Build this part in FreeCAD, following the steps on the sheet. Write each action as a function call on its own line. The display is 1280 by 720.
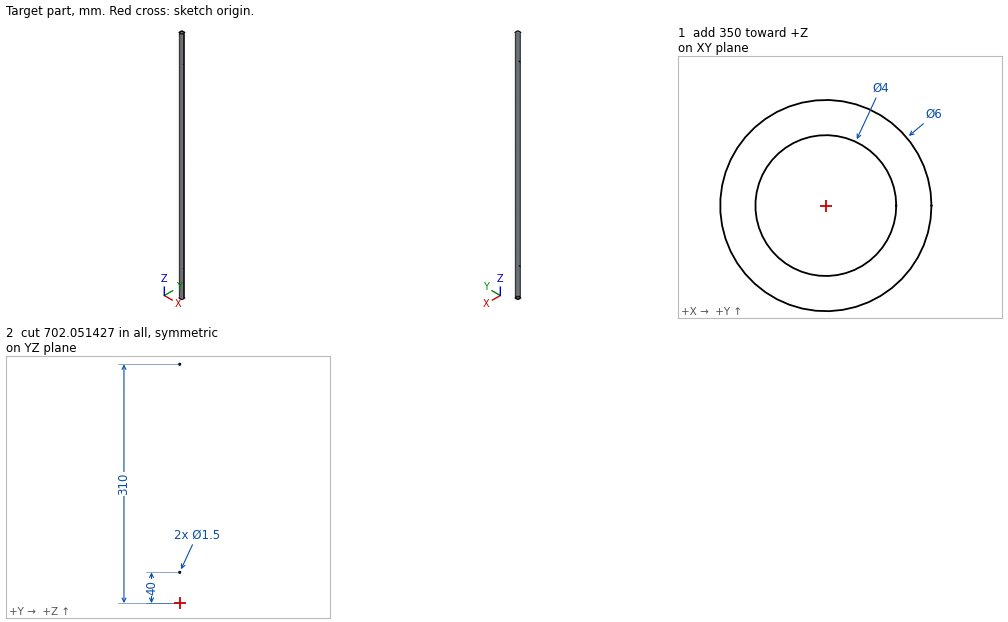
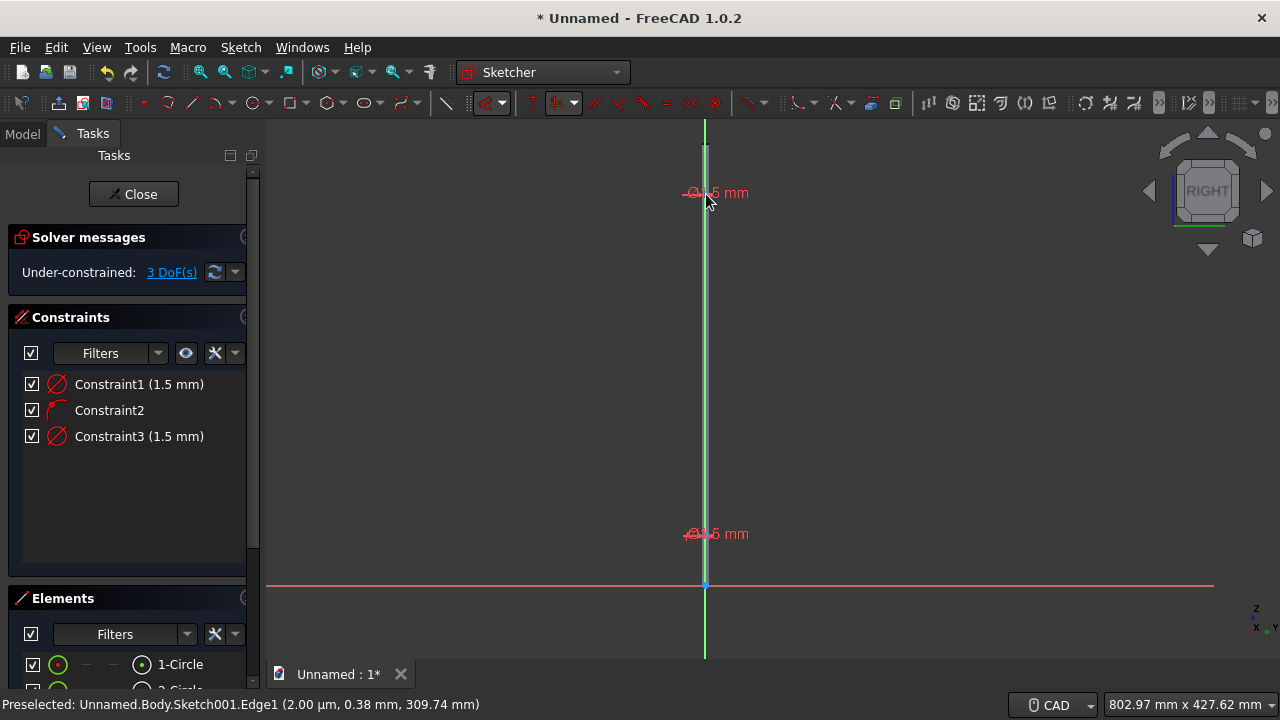
click(705, 195)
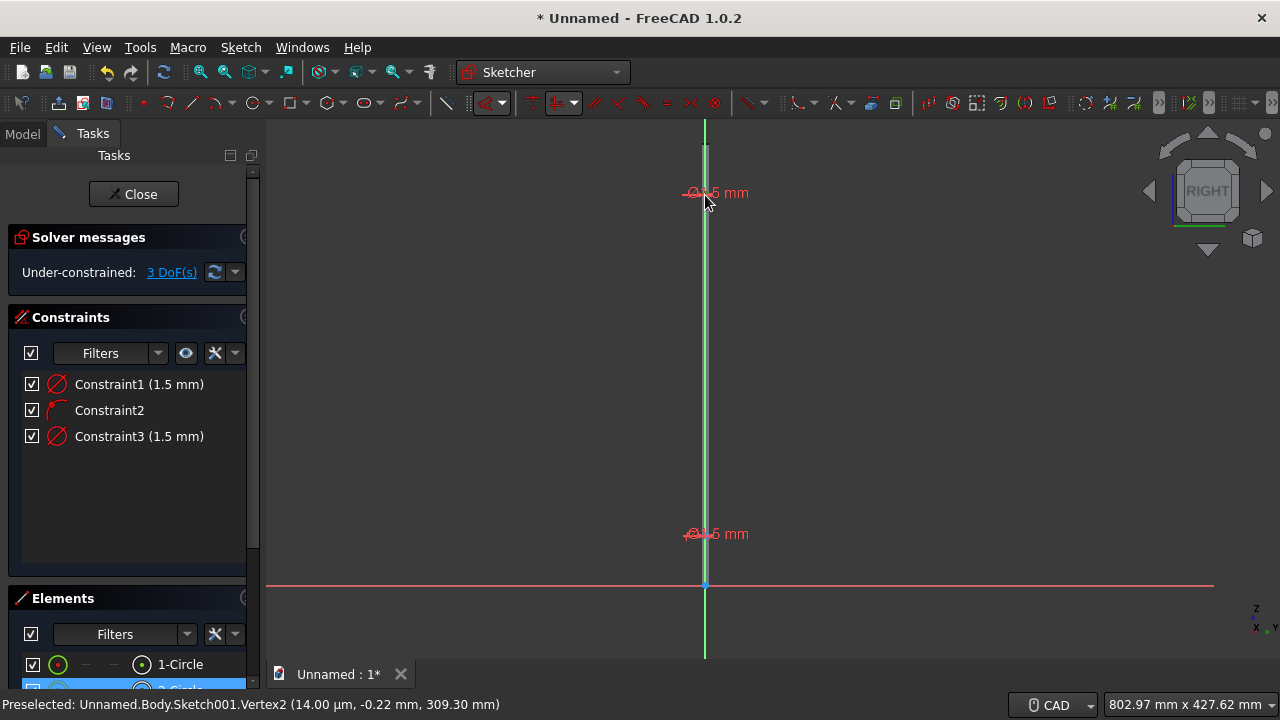
click(705, 493)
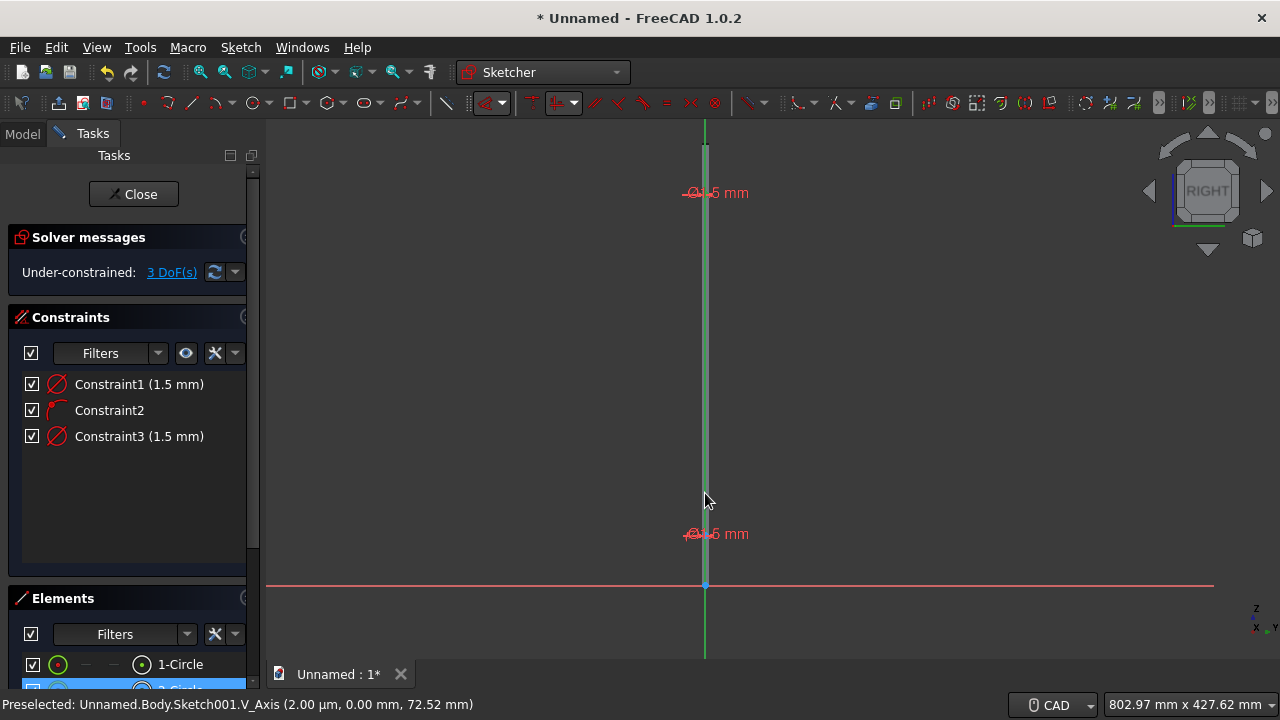
key(c)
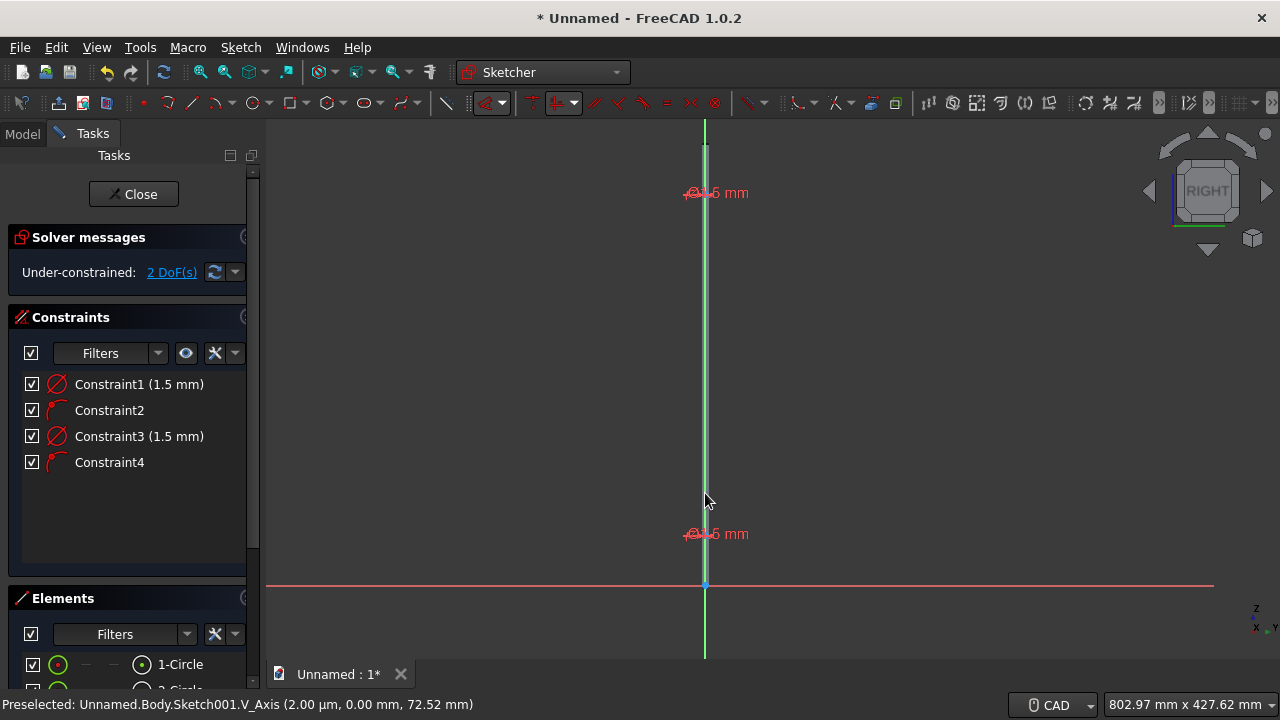
click(486, 104)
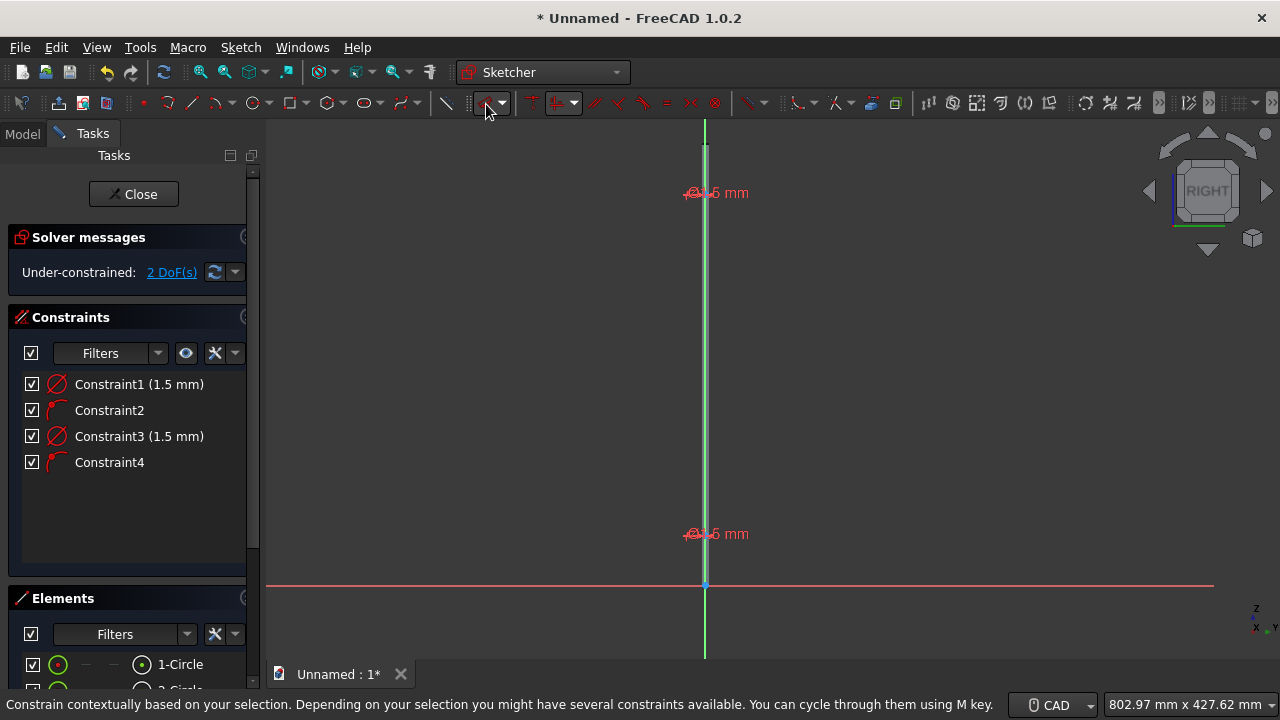
click(705, 536)
click(739, 561)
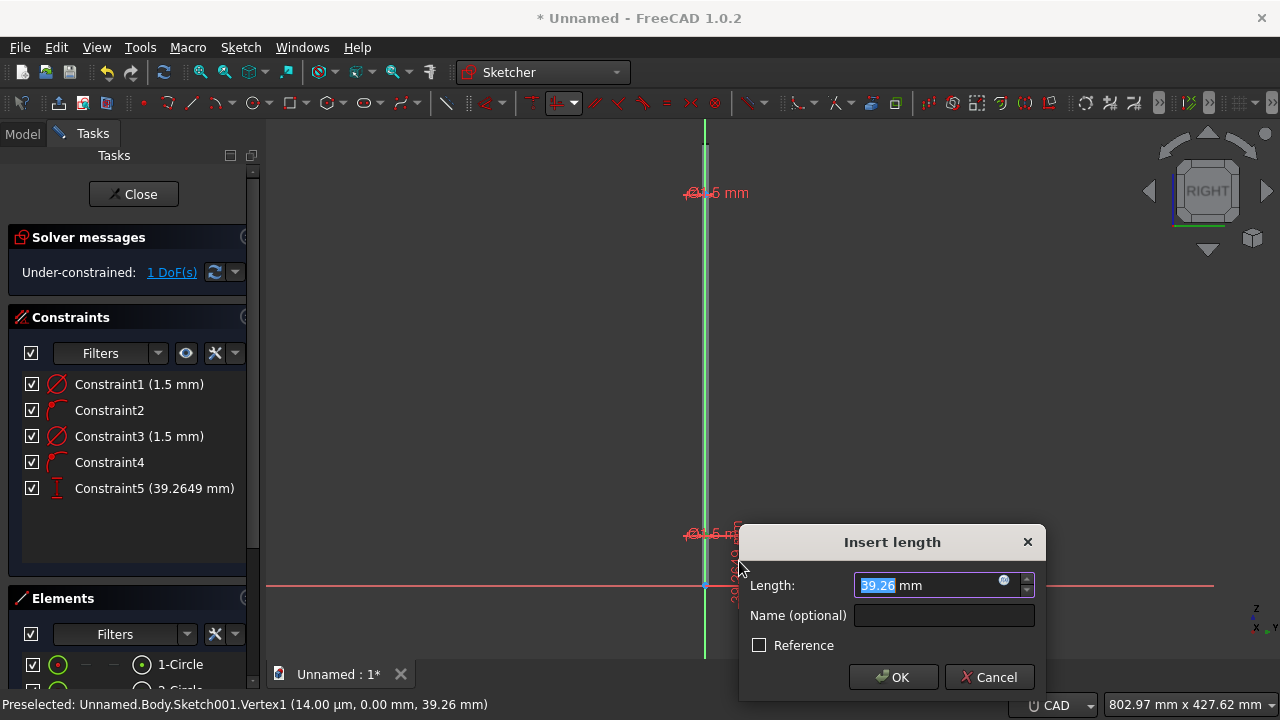
text(40)
key(Return)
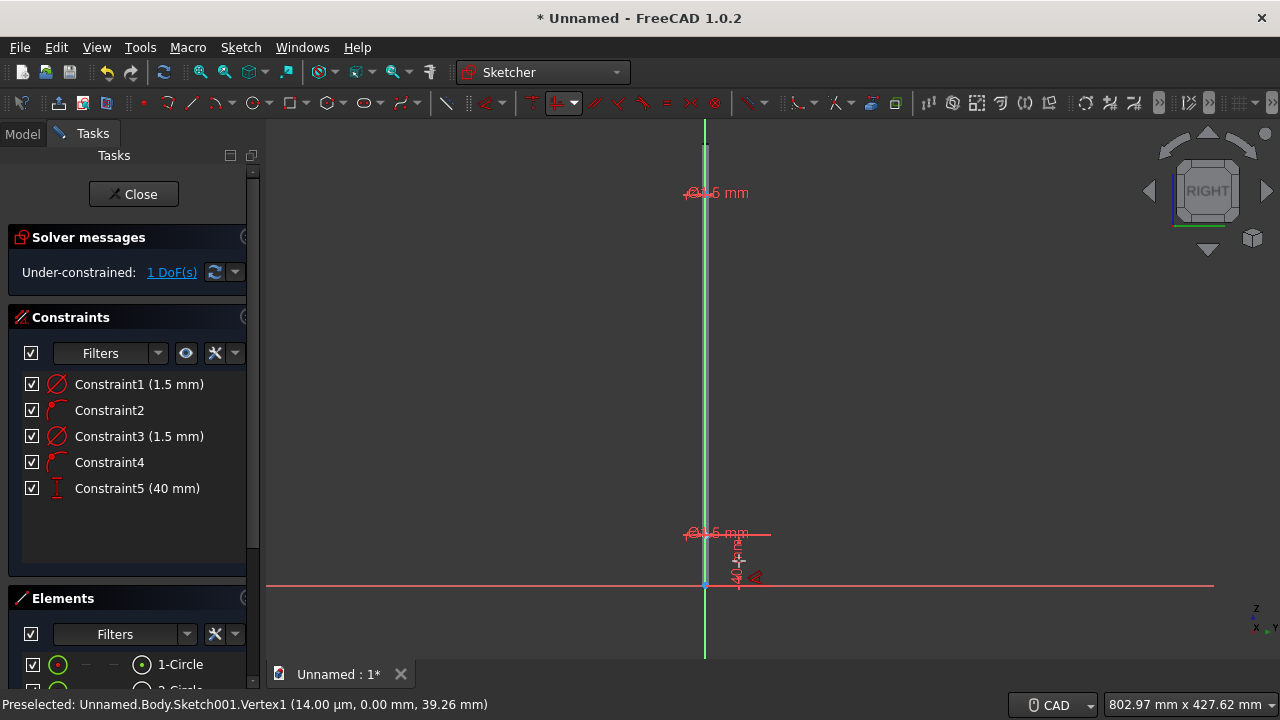
click(705, 195)
click(739, 390)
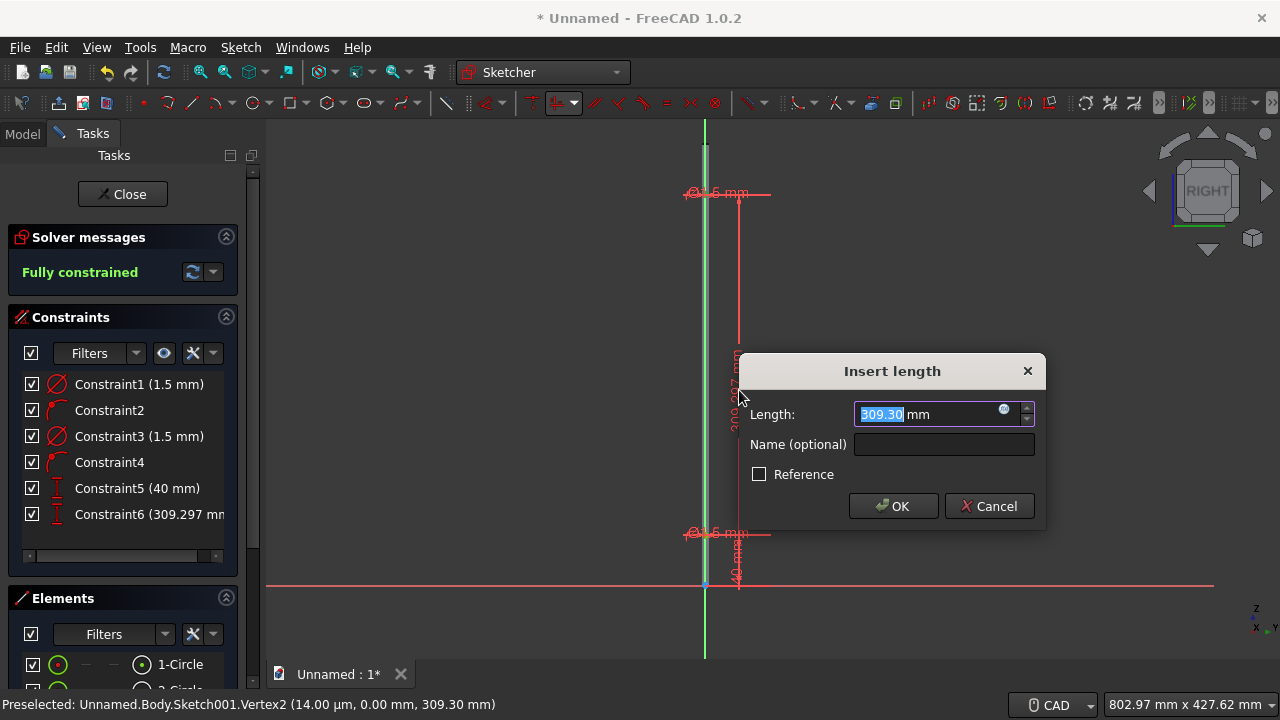
text(310)
key(Return)
key(Escape)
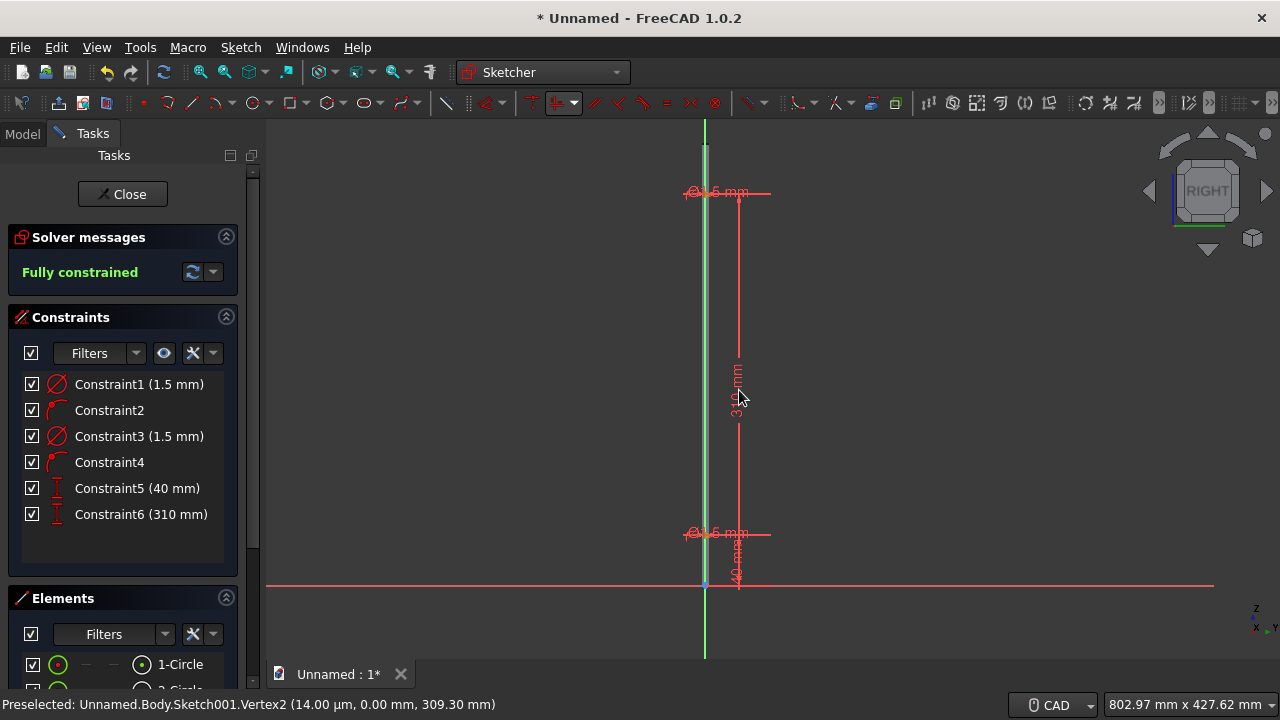
click(123, 194)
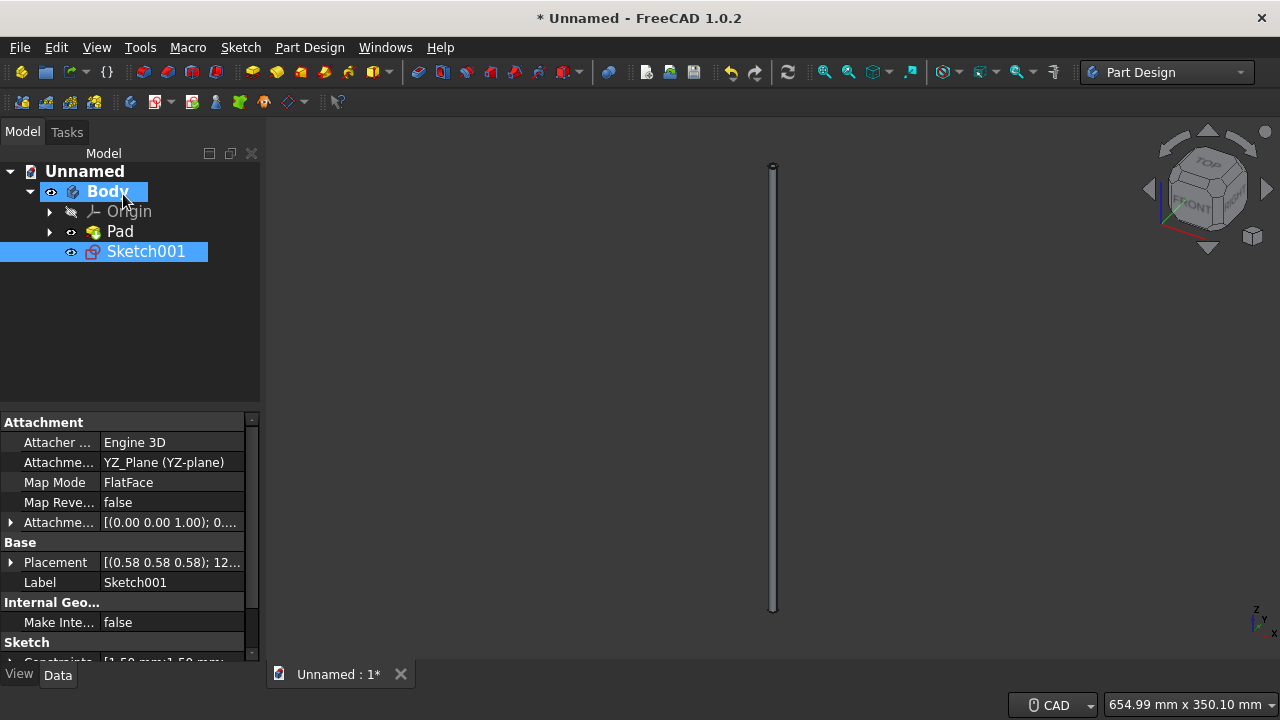
click(420, 72)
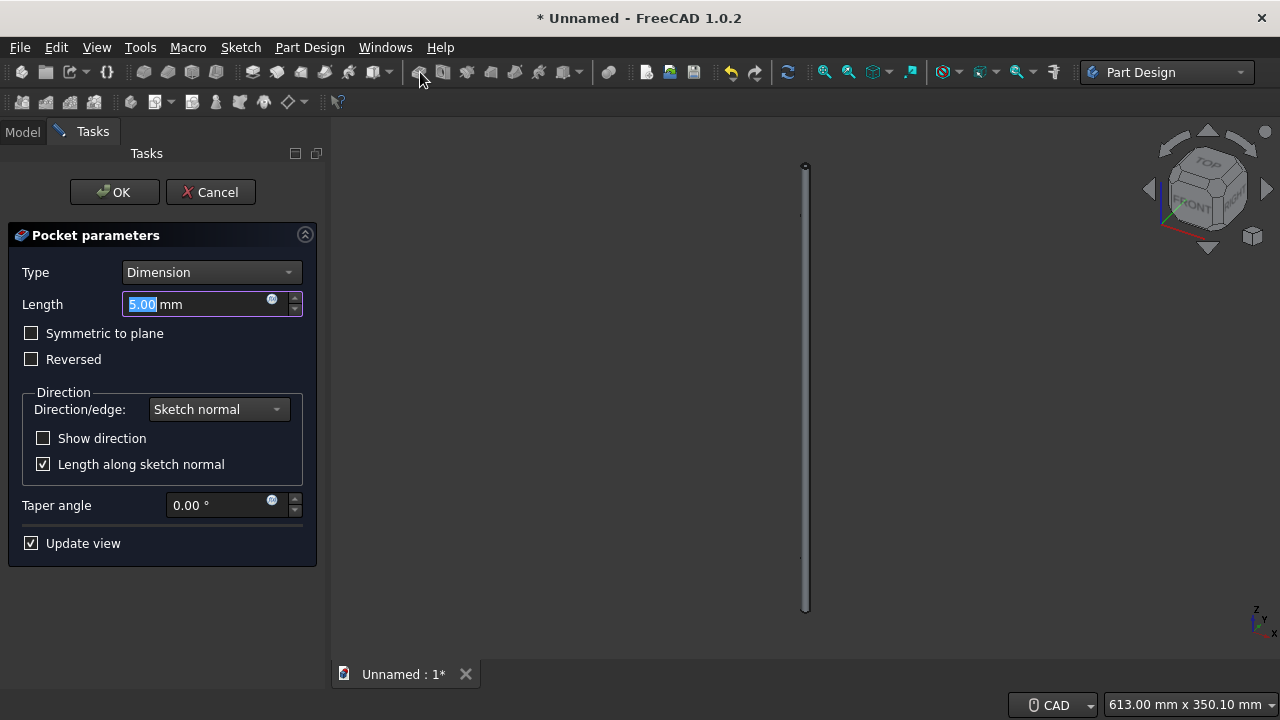
text(702.051427)
key(Tab)